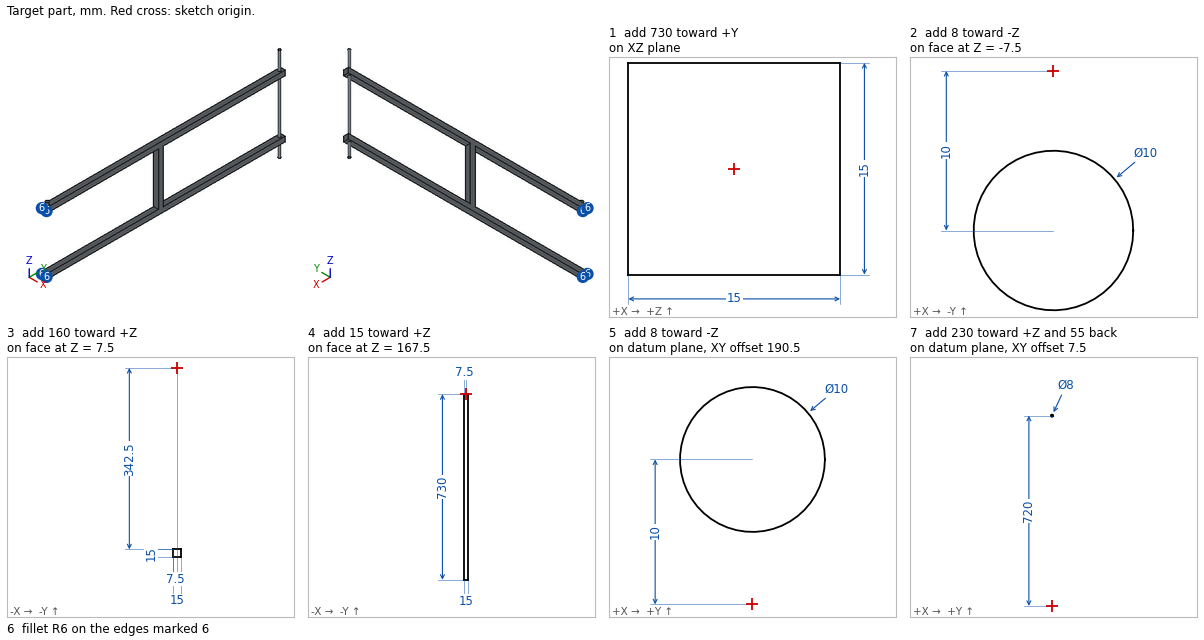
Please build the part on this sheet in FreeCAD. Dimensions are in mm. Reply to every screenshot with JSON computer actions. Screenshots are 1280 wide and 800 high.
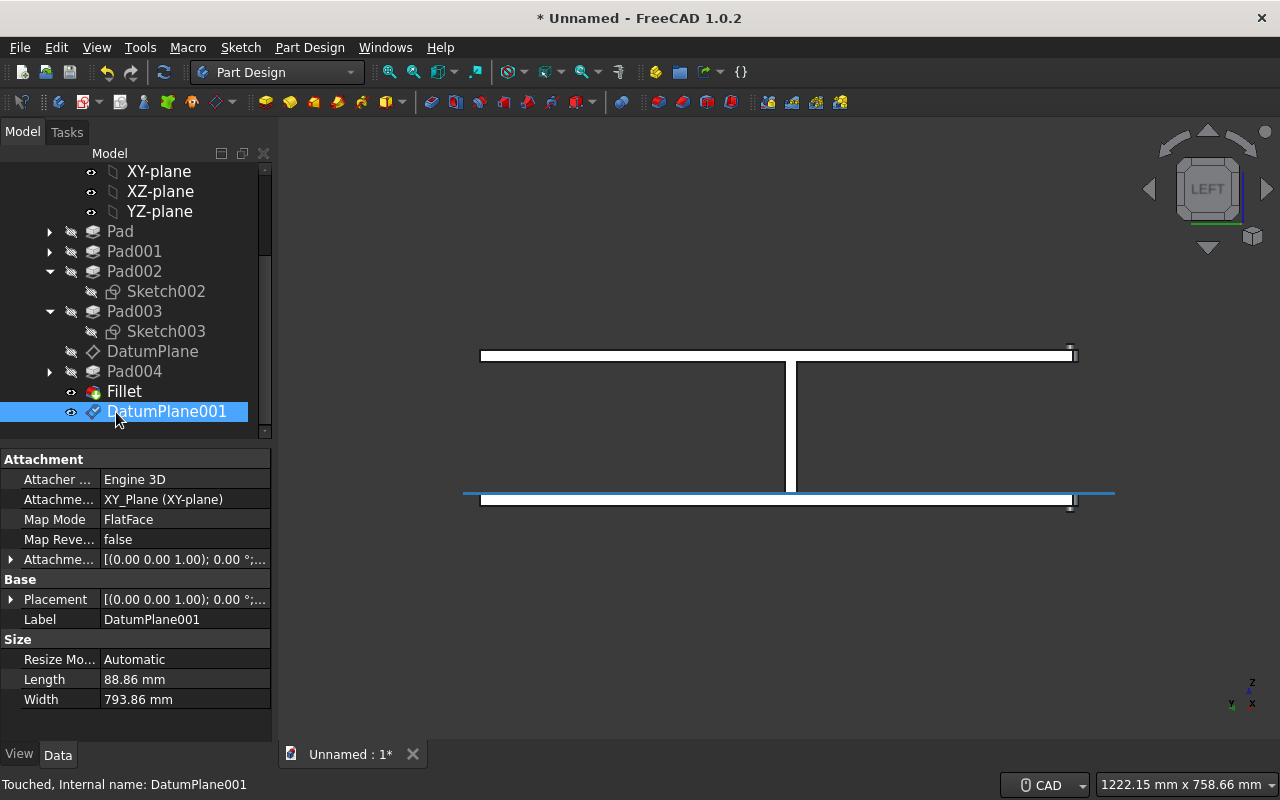
{"action": "left_click", "coordinate": [84, 102]}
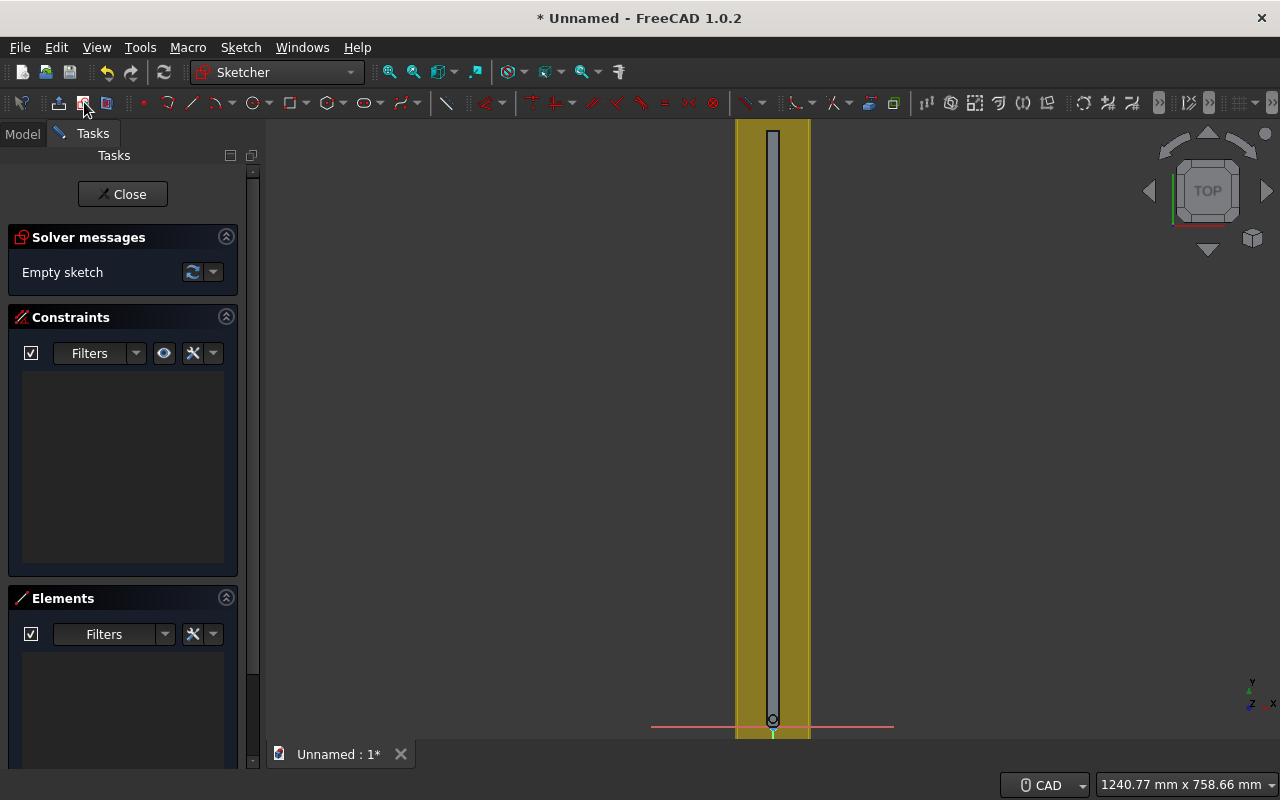
{"action": "left_click", "coordinate": [108, 104]}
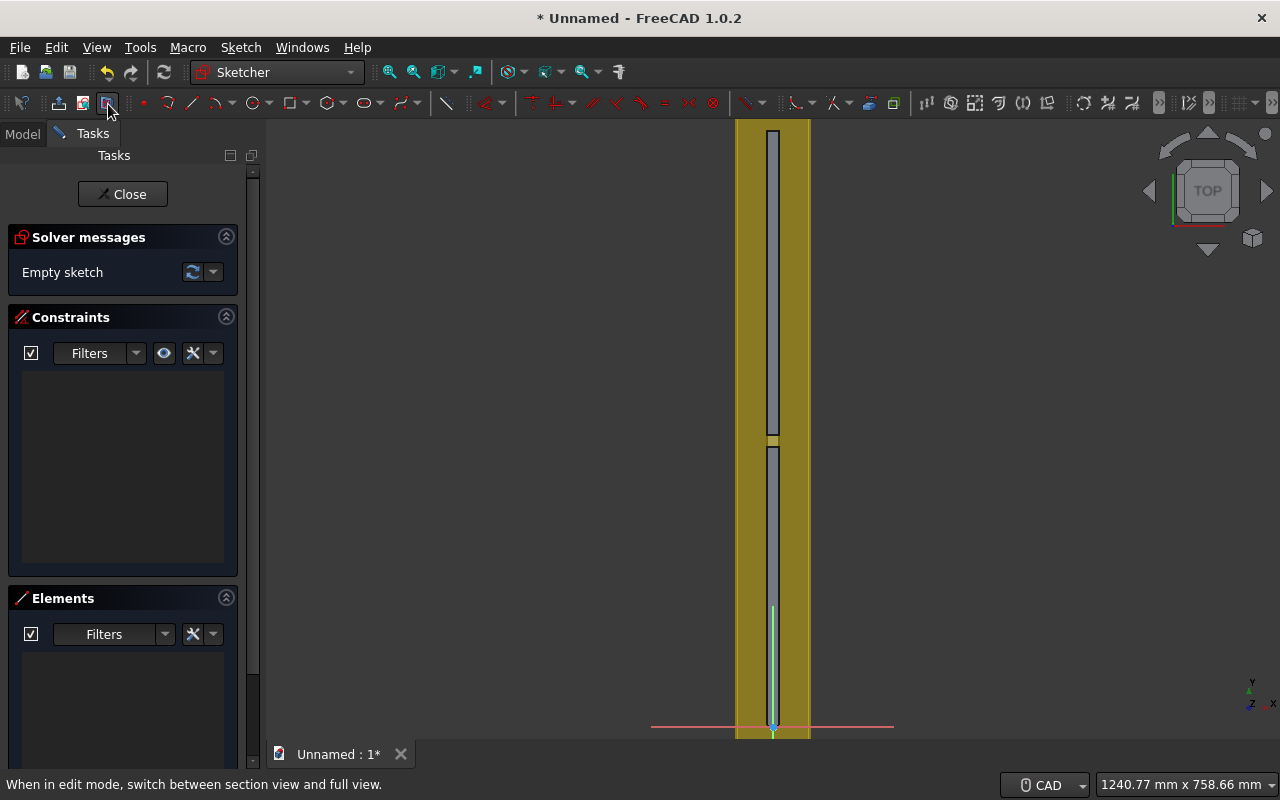
{"action": "scroll", "coordinate": [704, 429], "scroll_direction": "down", "scroll_amount": 5}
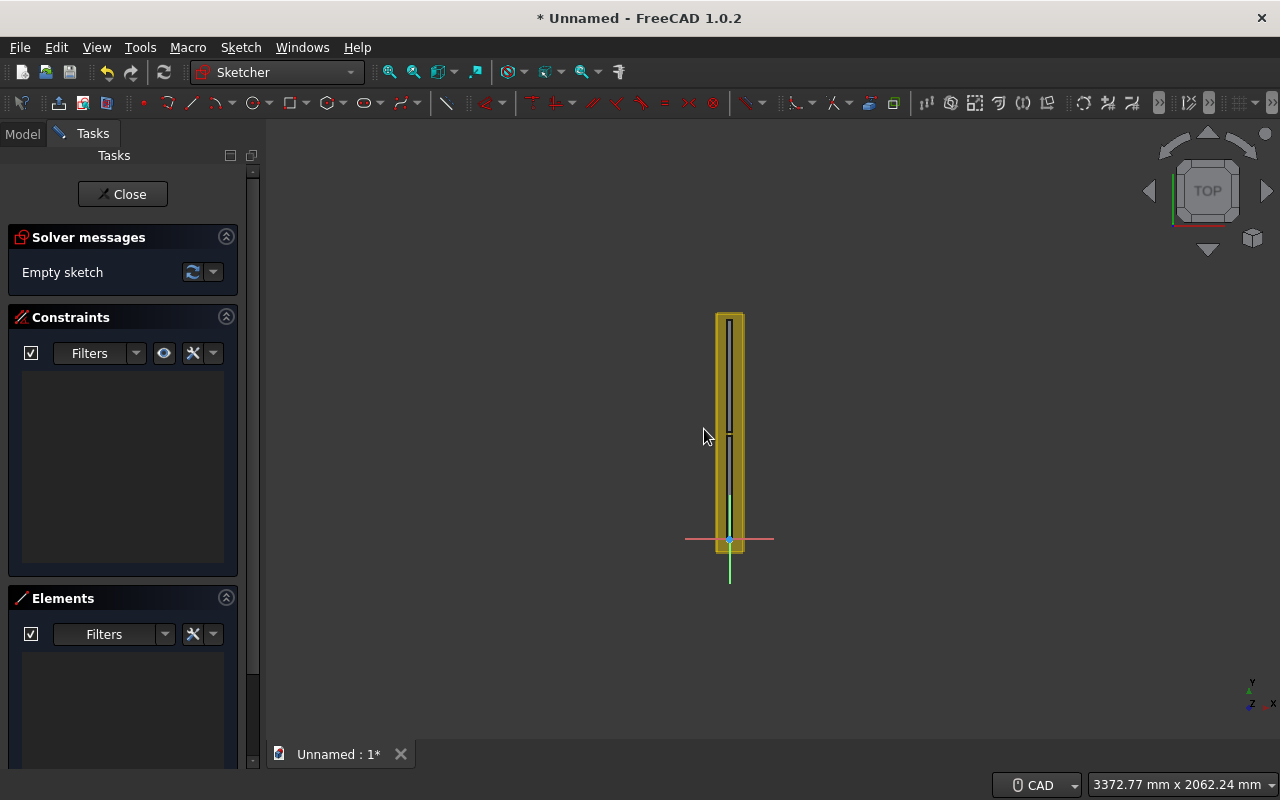
{"action": "scroll", "coordinate": [731, 317], "scroll_direction": "up", "scroll_amount": 15}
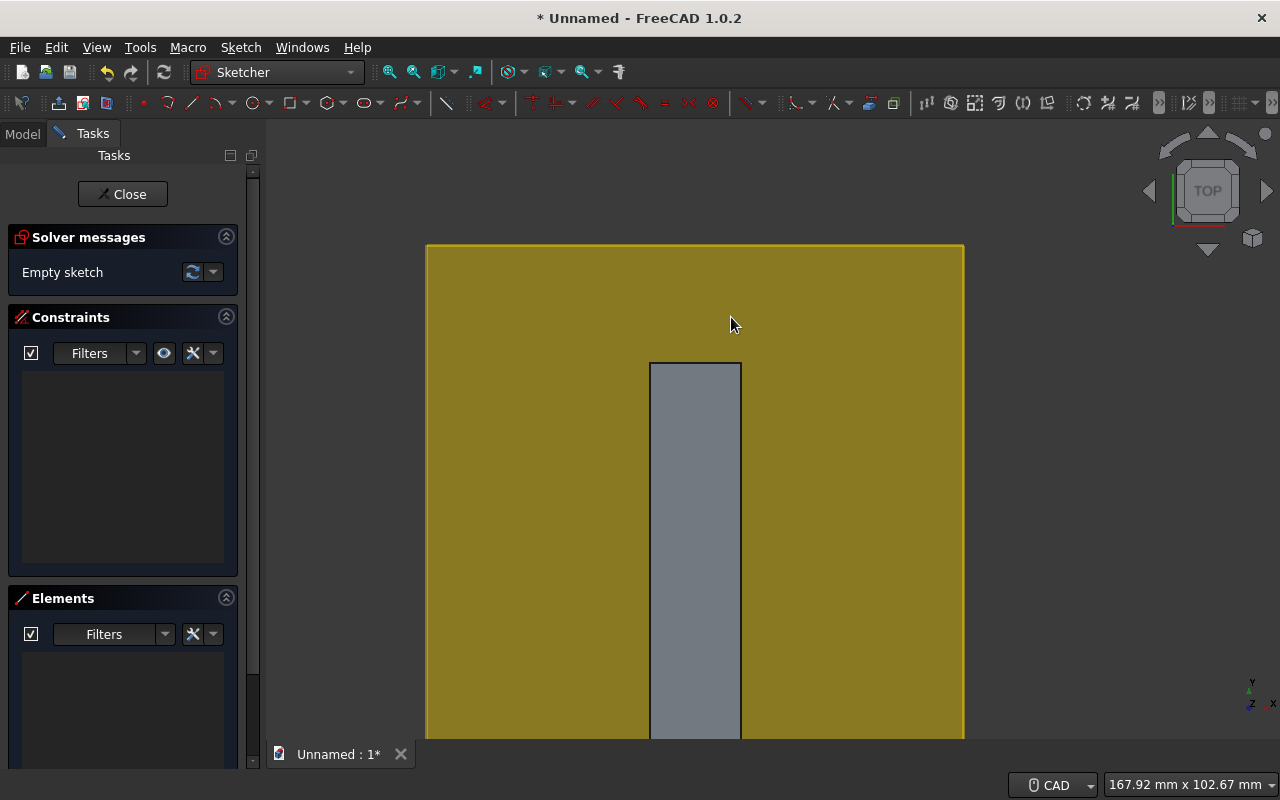
{"action": "scroll", "coordinate": [694, 422], "scroll_direction": "up", "scroll_amount": 11}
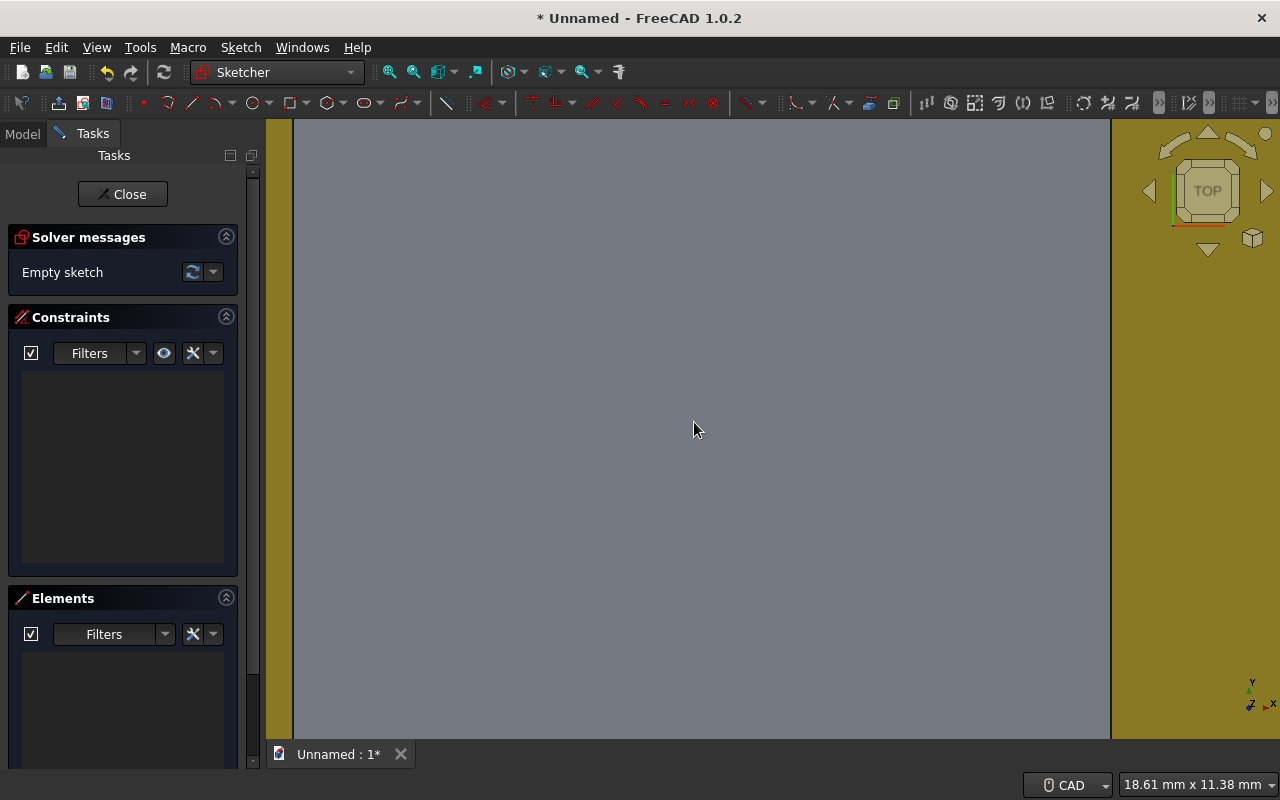
{"action": "left_click", "coordinate": [254, 104]}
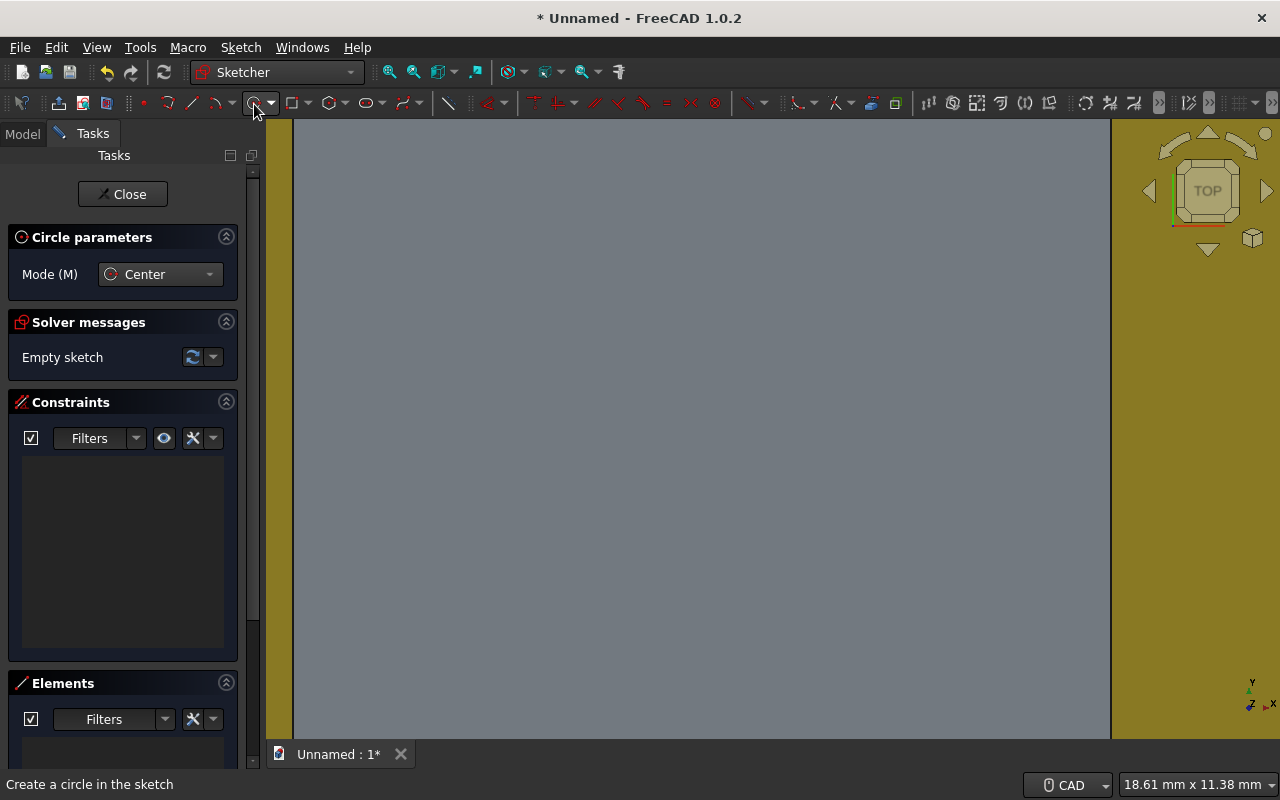
{"action": "left_click", "coordinate": [702, 428]}
{"action": "left_click", "coordinate": [856, 274]}
{"action": "key", "text": "Escape"}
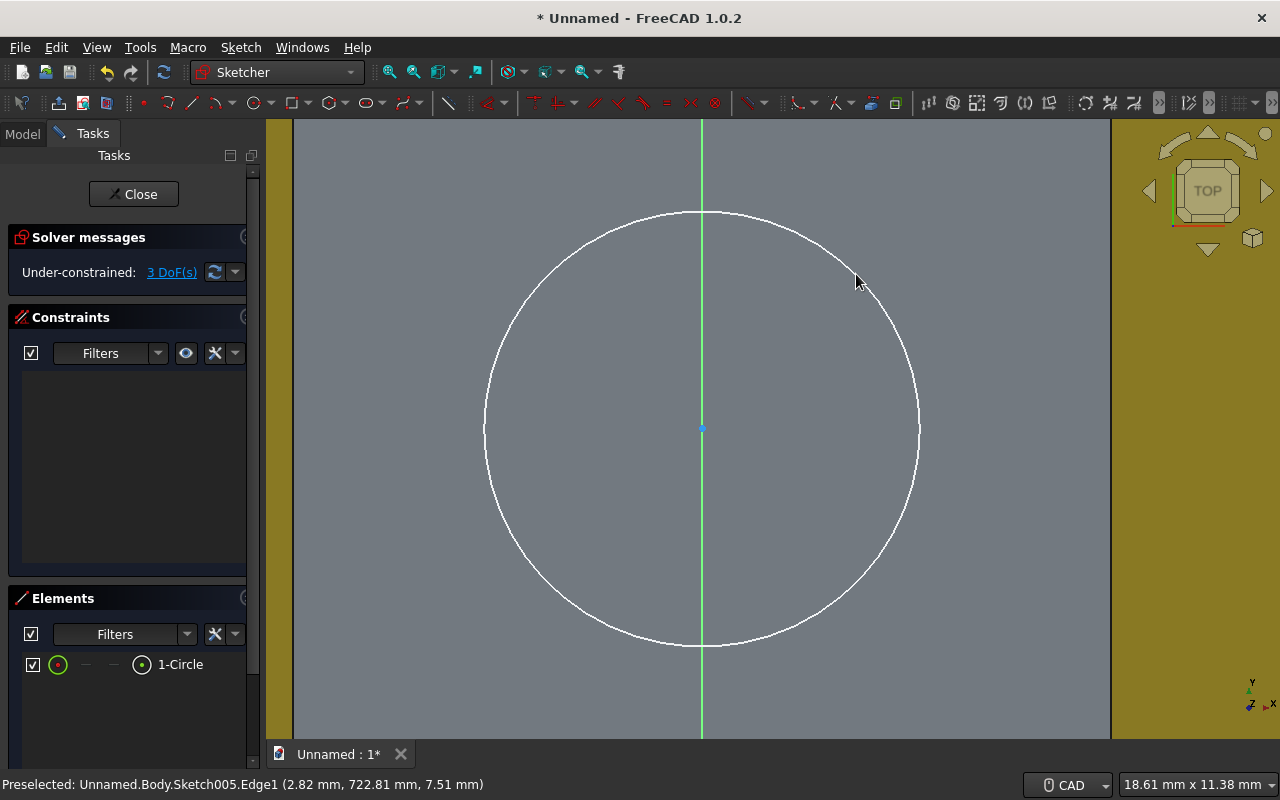
{"action": "left_click", "coordinate": [702, 429]}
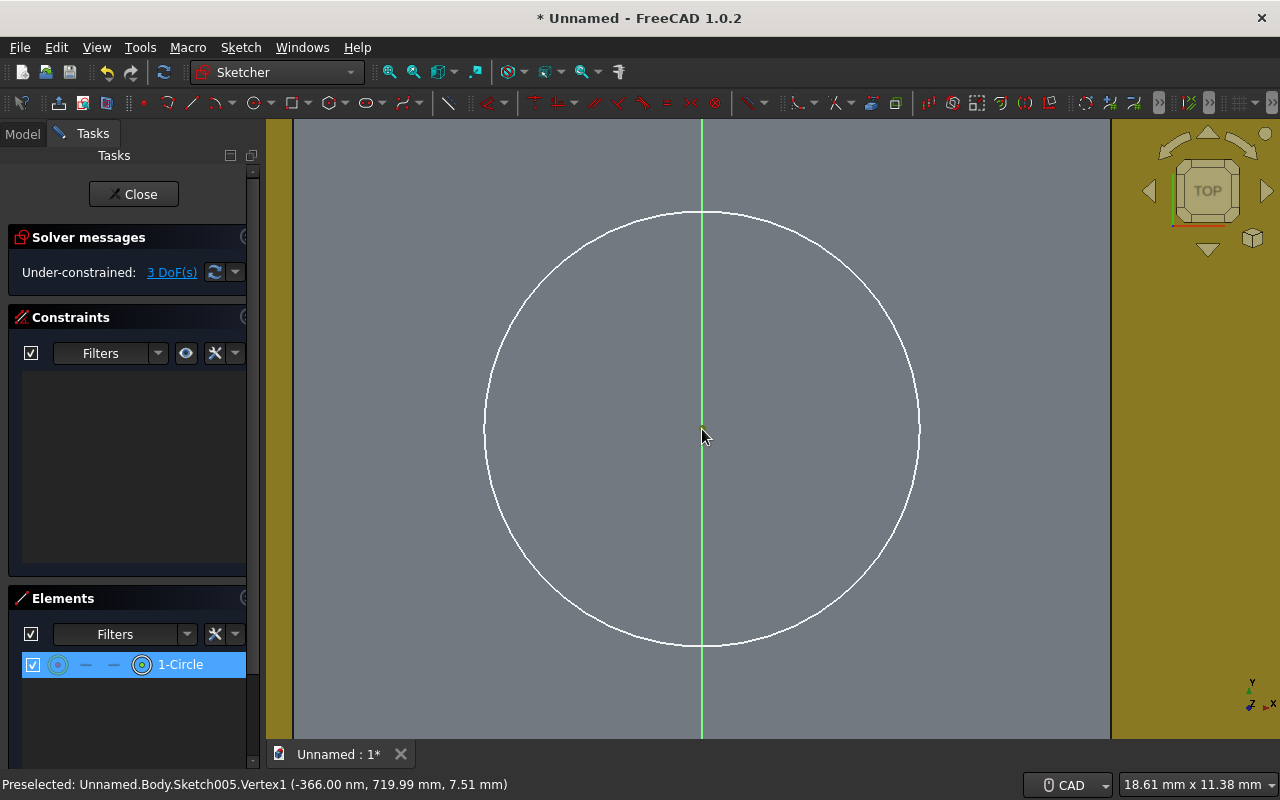
{"action": "left_click", "coordinate": [702, 590]}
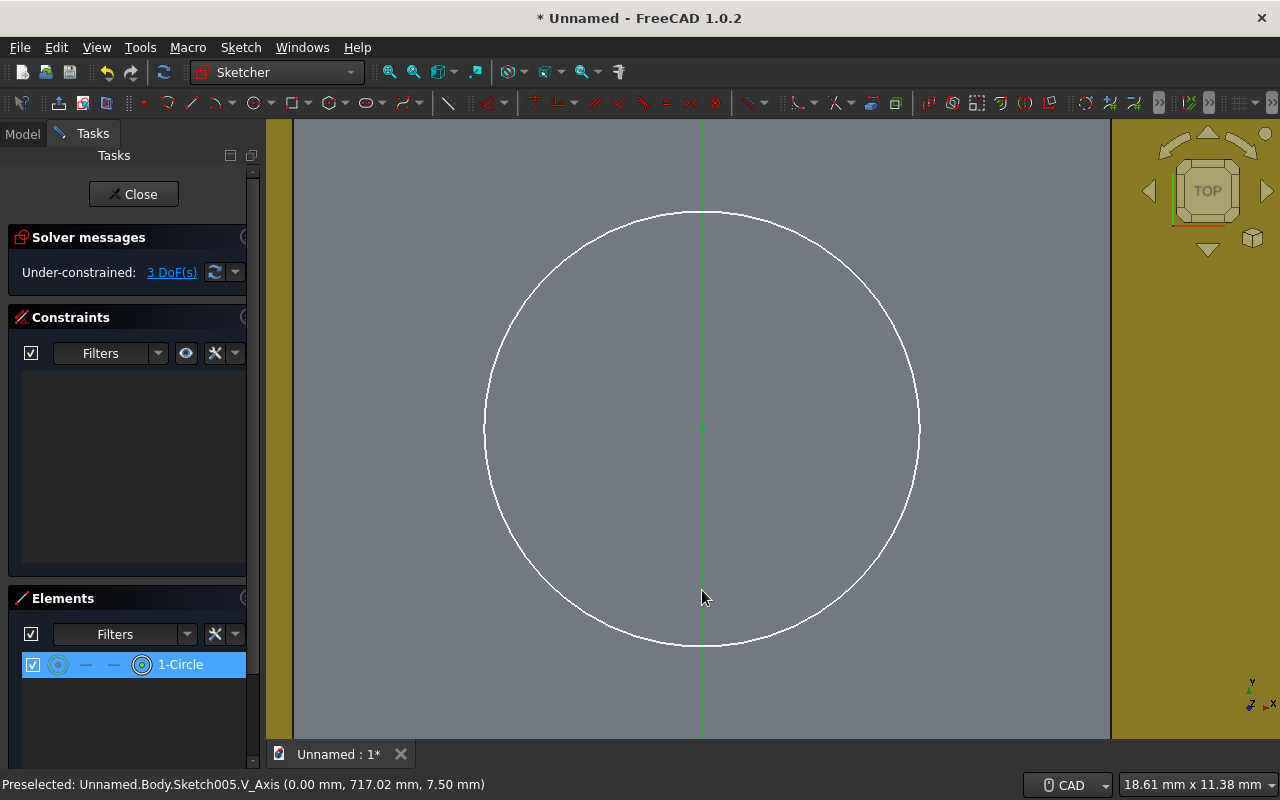
{"action": "left_click", "coordinate": [534, 104]}